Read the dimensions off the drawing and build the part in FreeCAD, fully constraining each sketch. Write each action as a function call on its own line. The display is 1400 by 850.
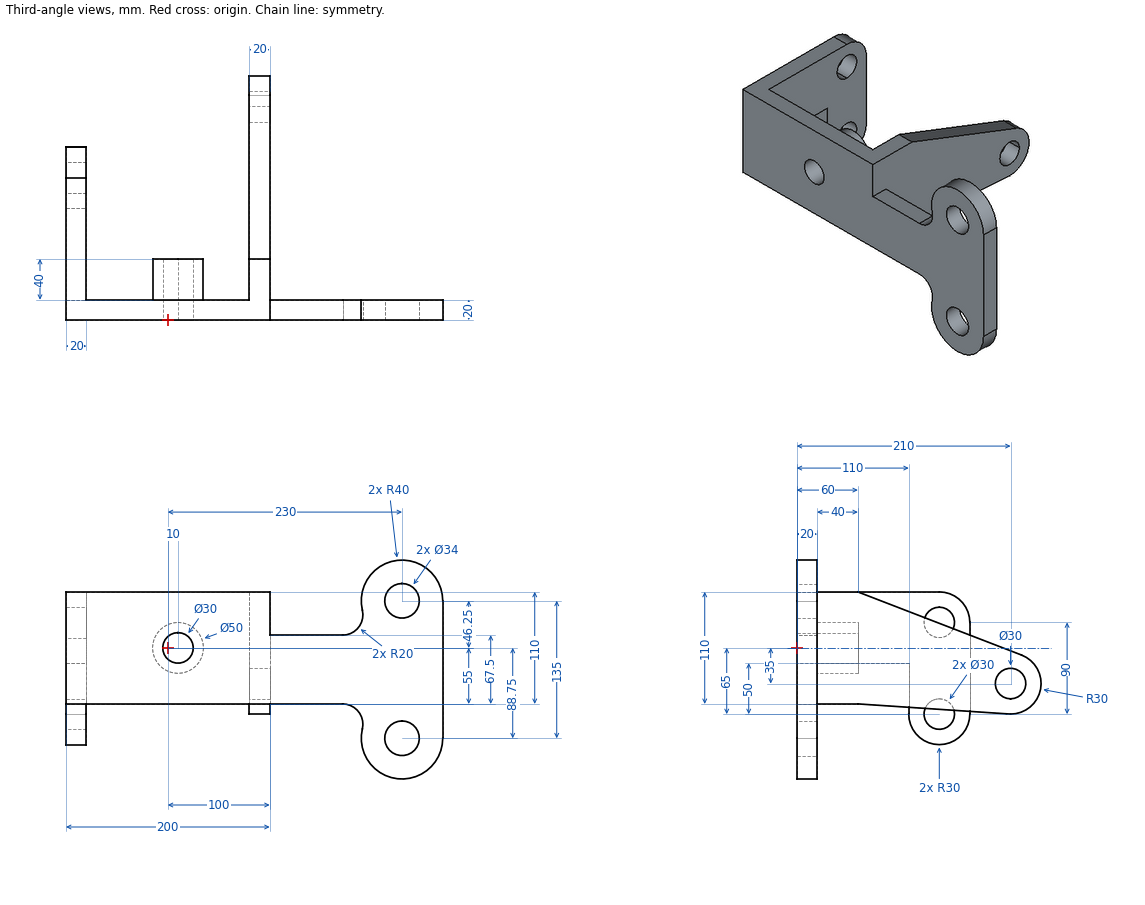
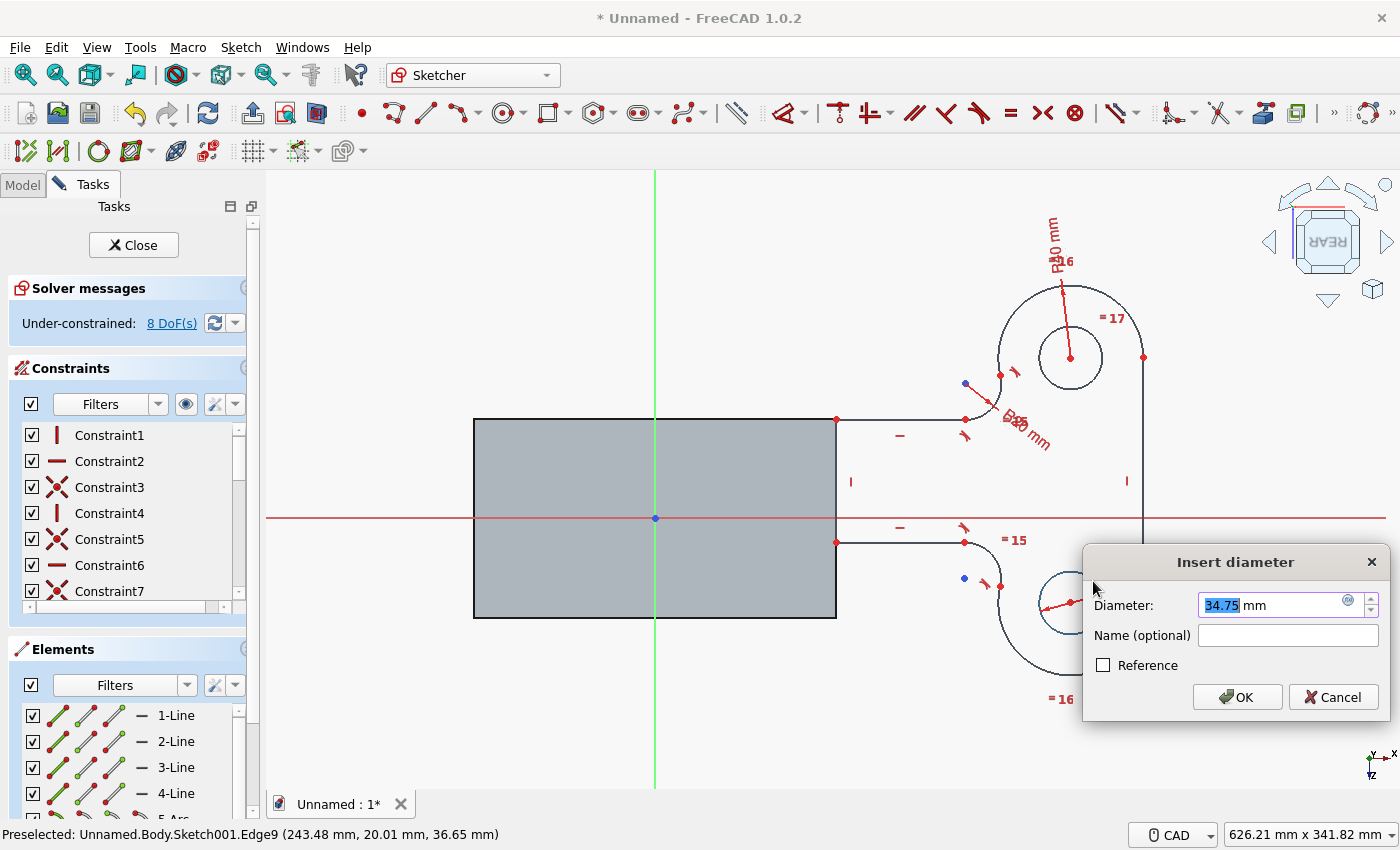
text(34)
key(Return)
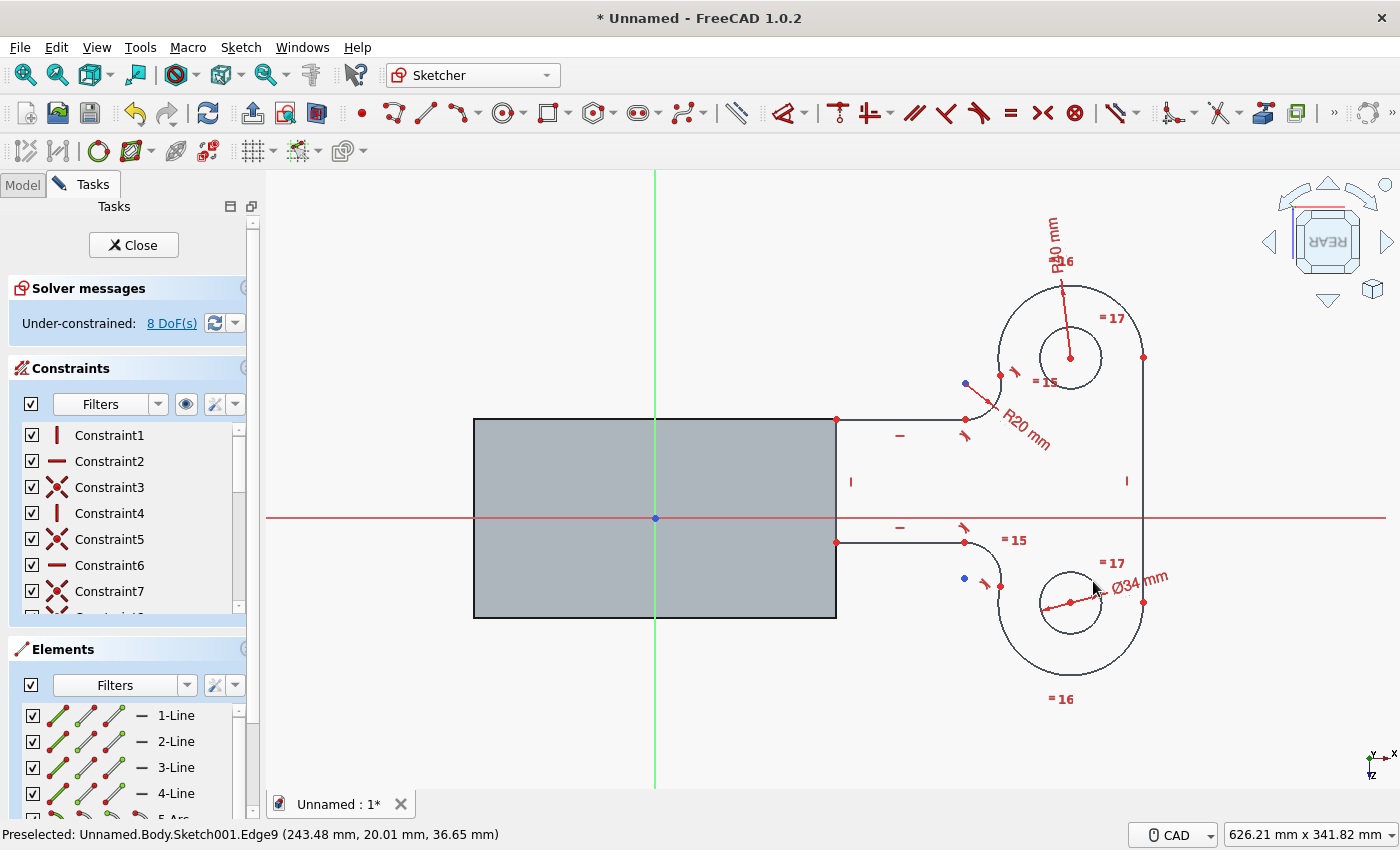
click(1143, 529)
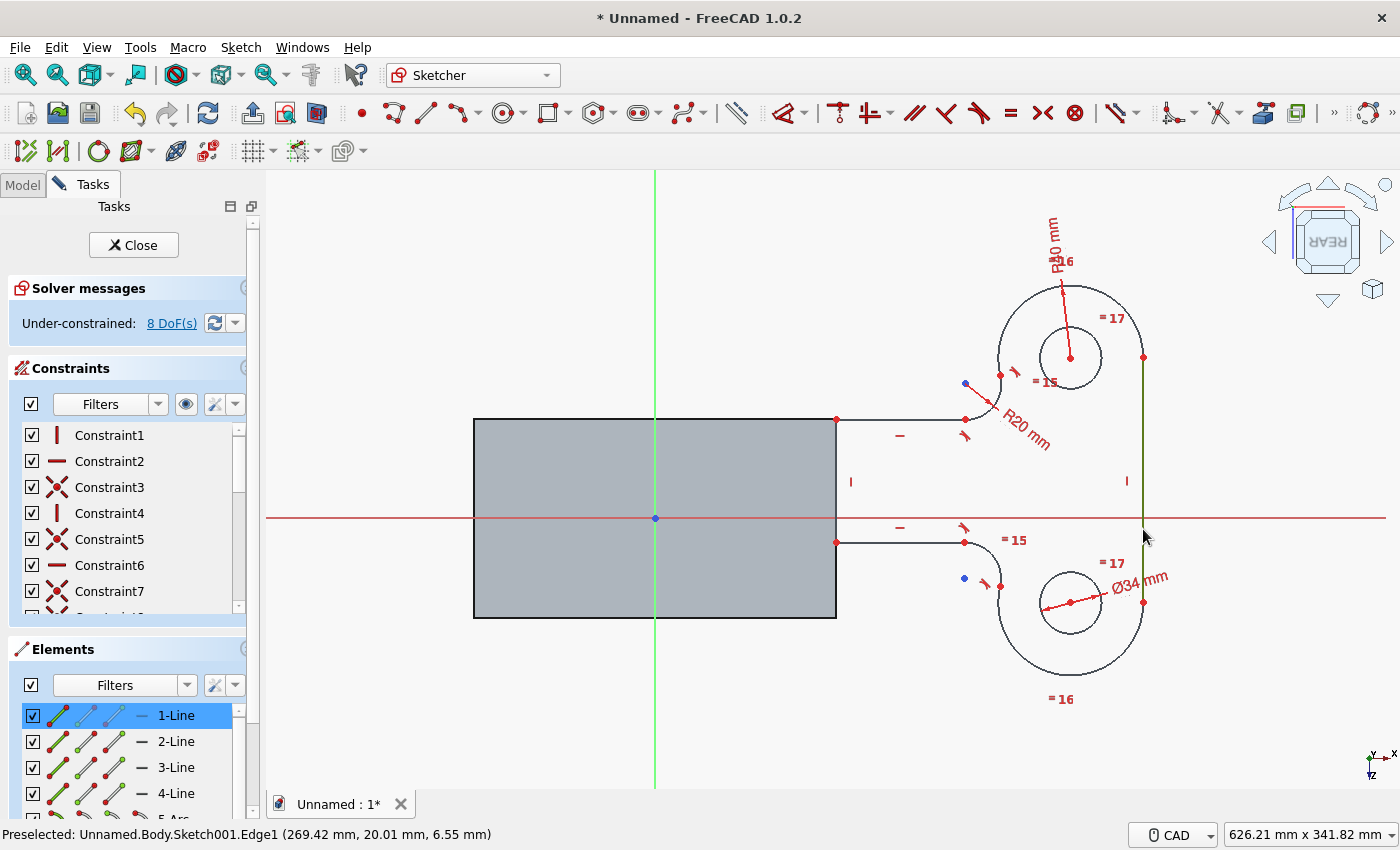
key(i)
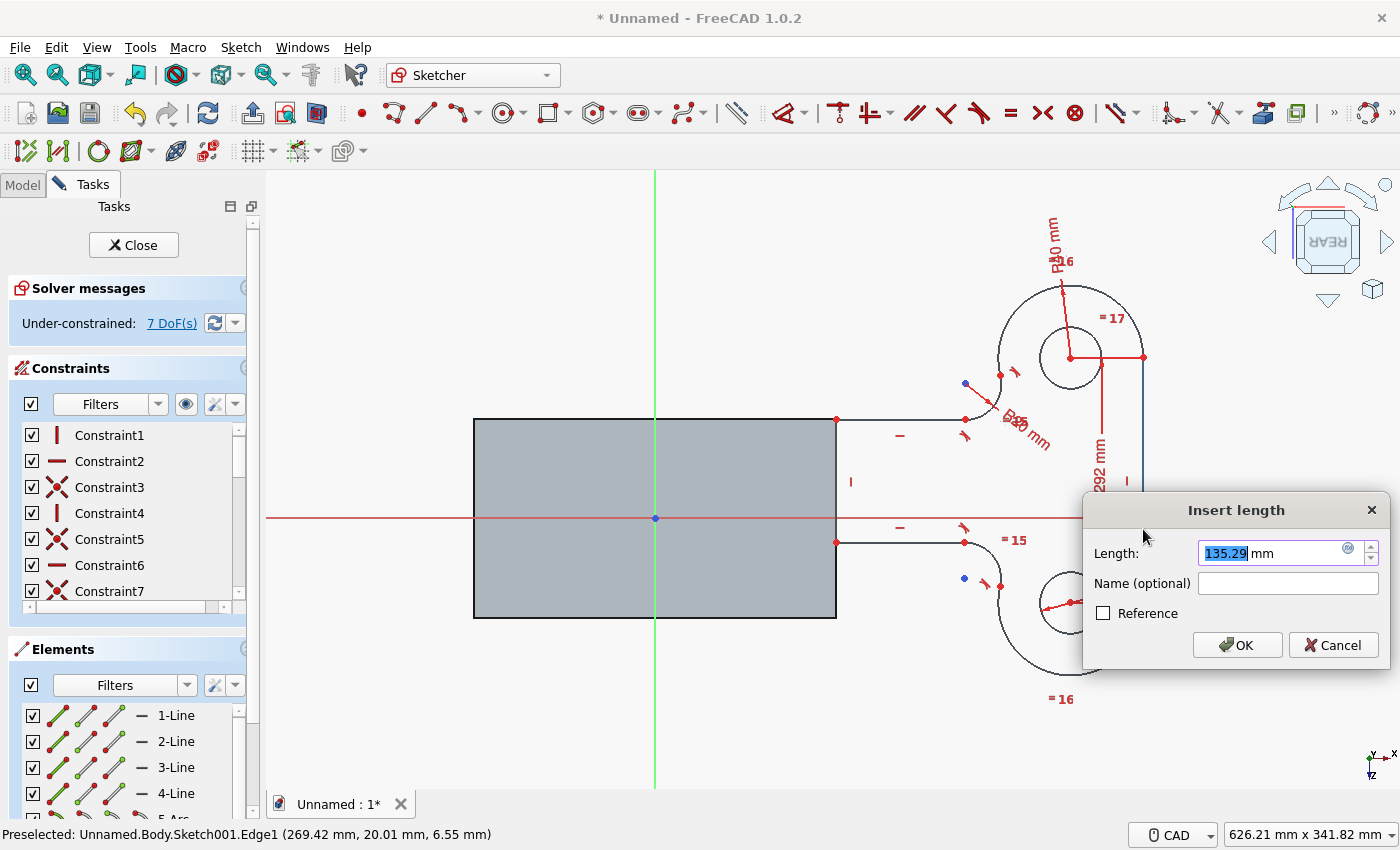
text(135)
key(Return)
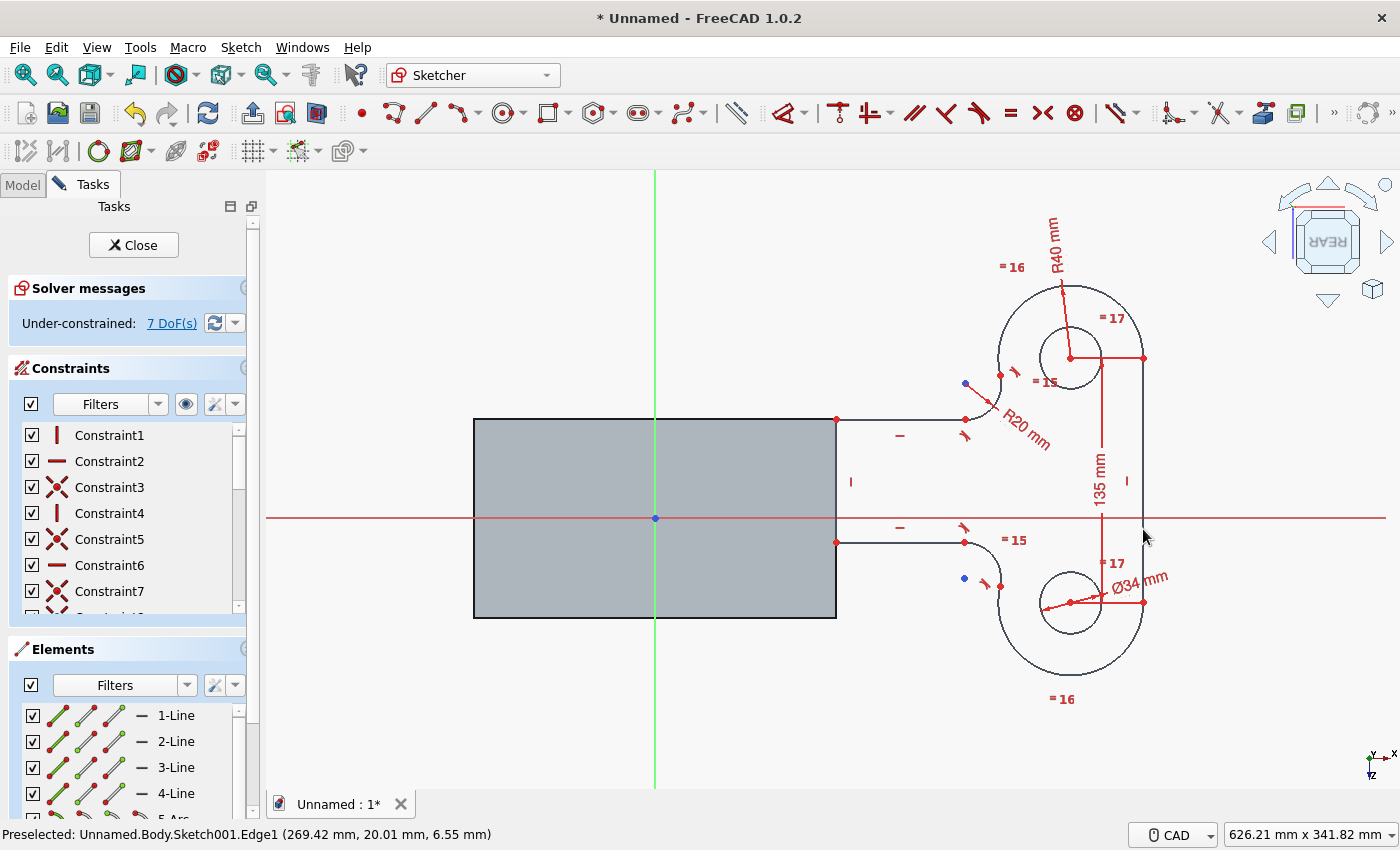
click(965, 420)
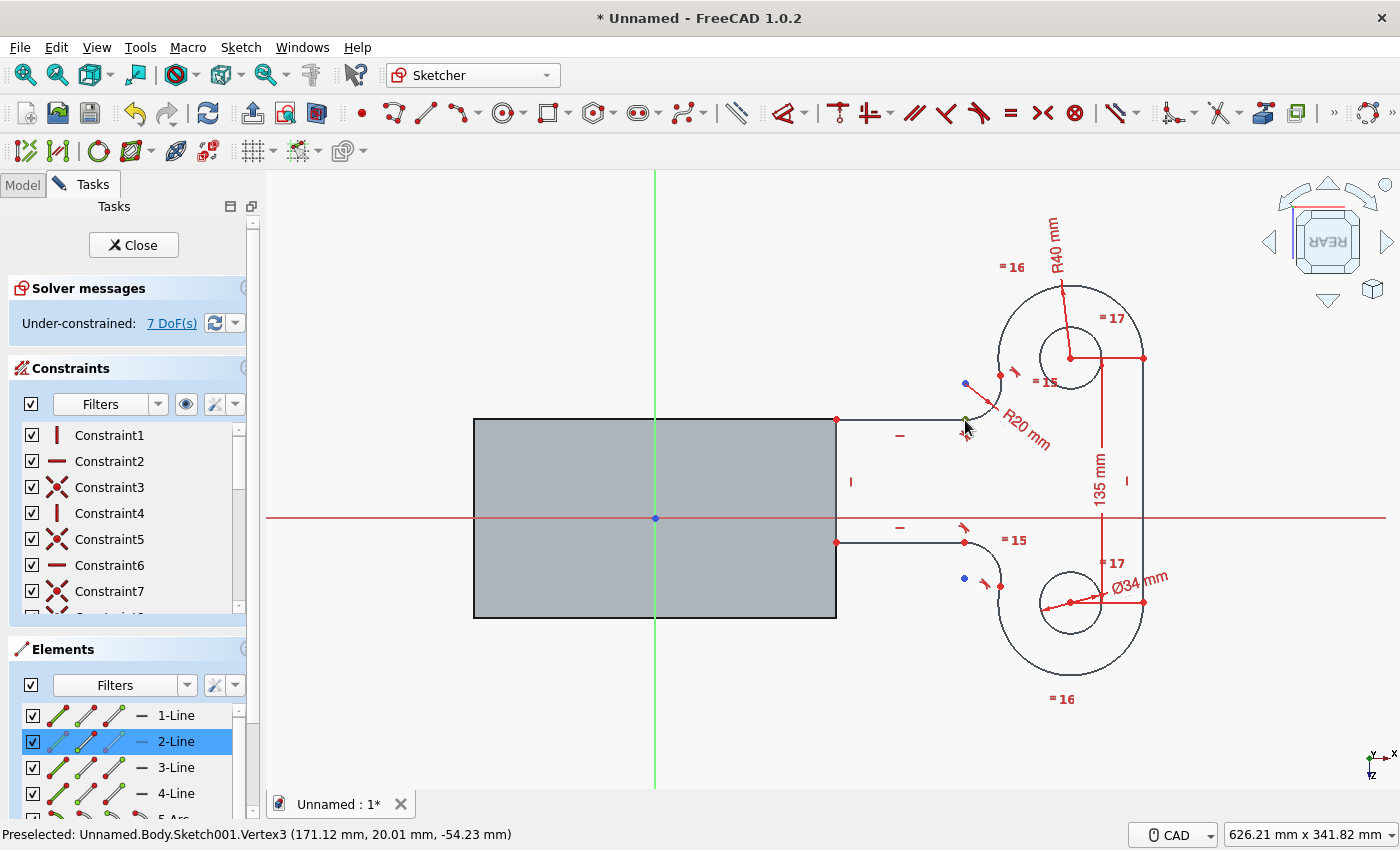
key(i)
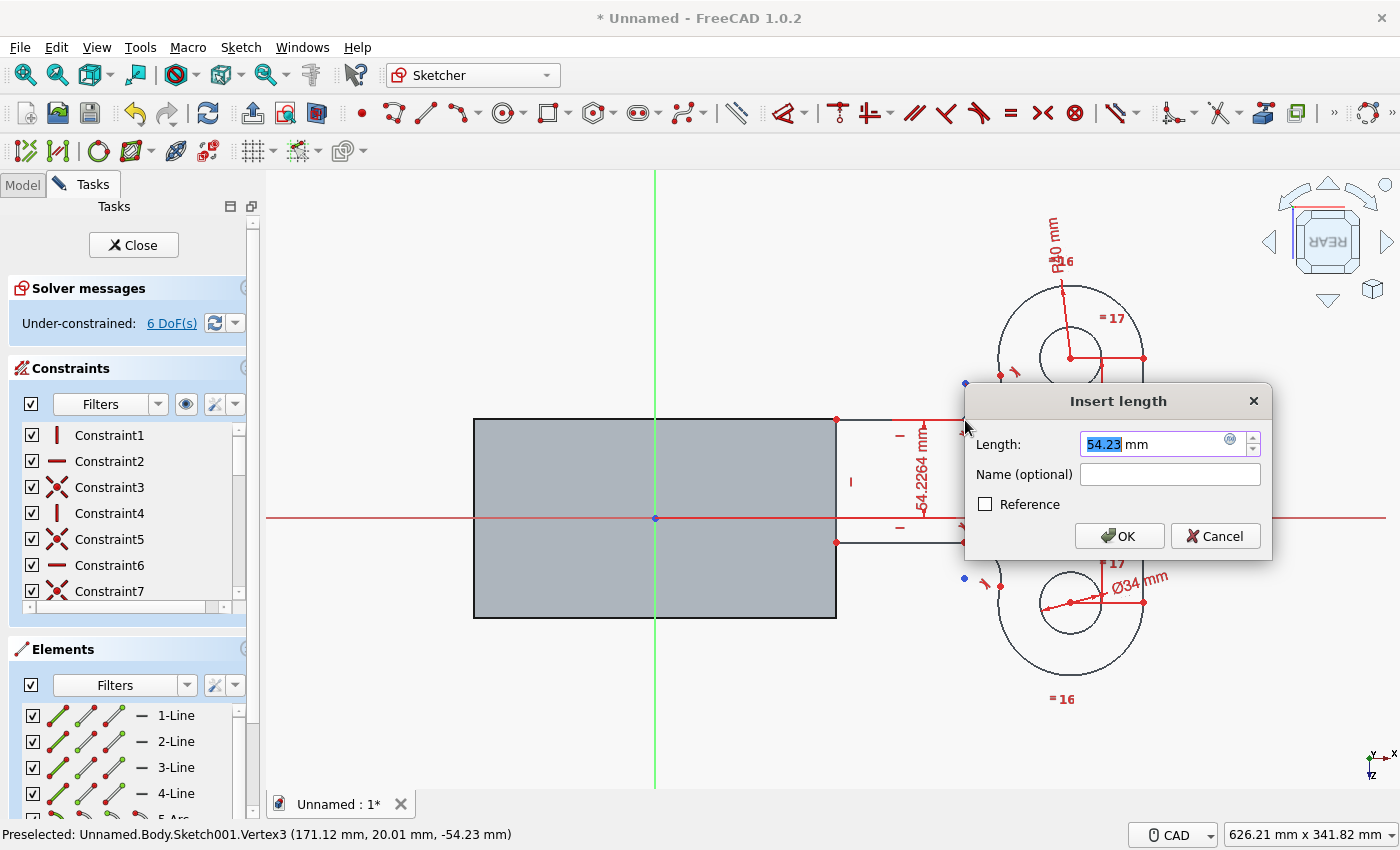
text(55)
key(Return)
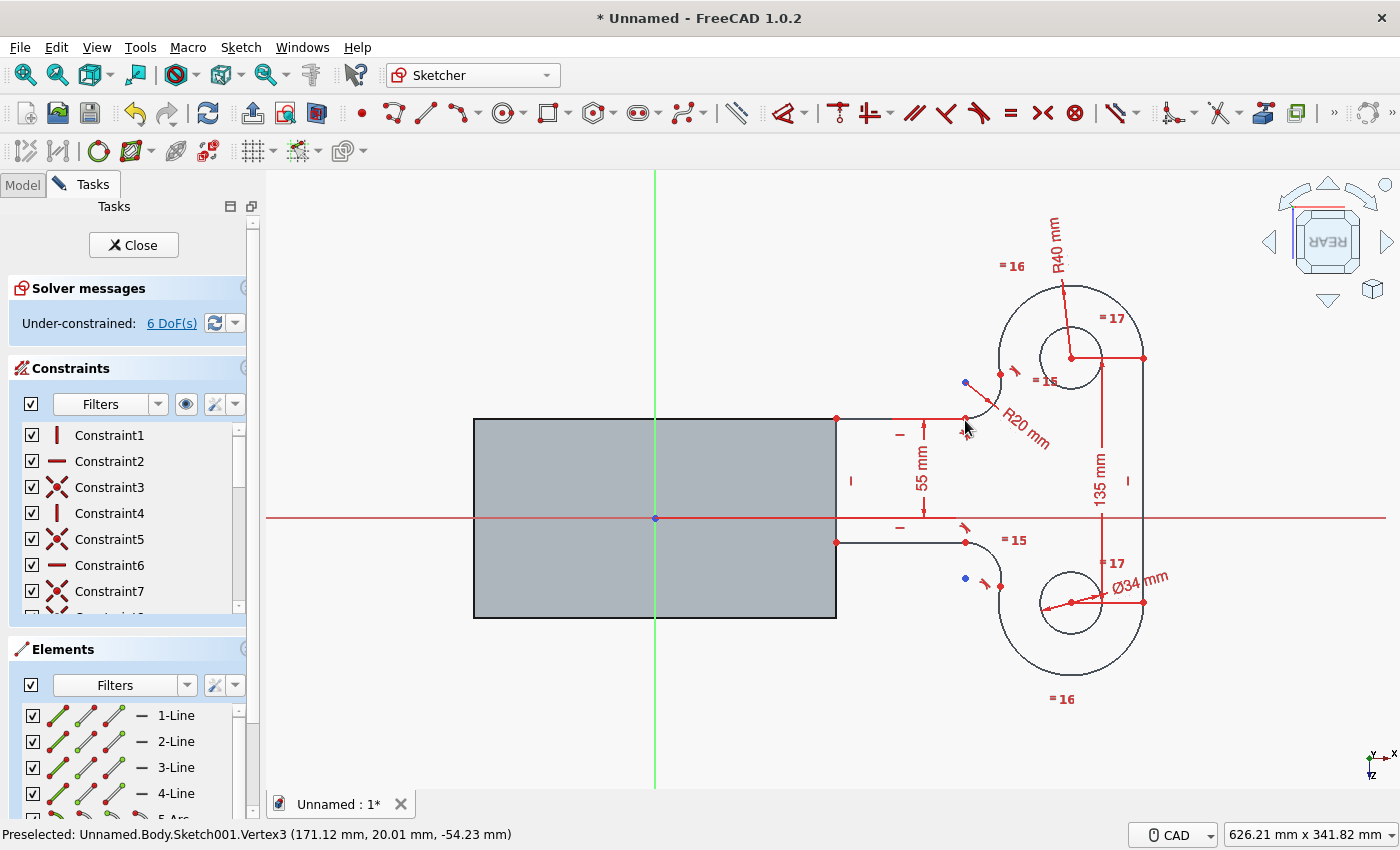
click(1071, 603)